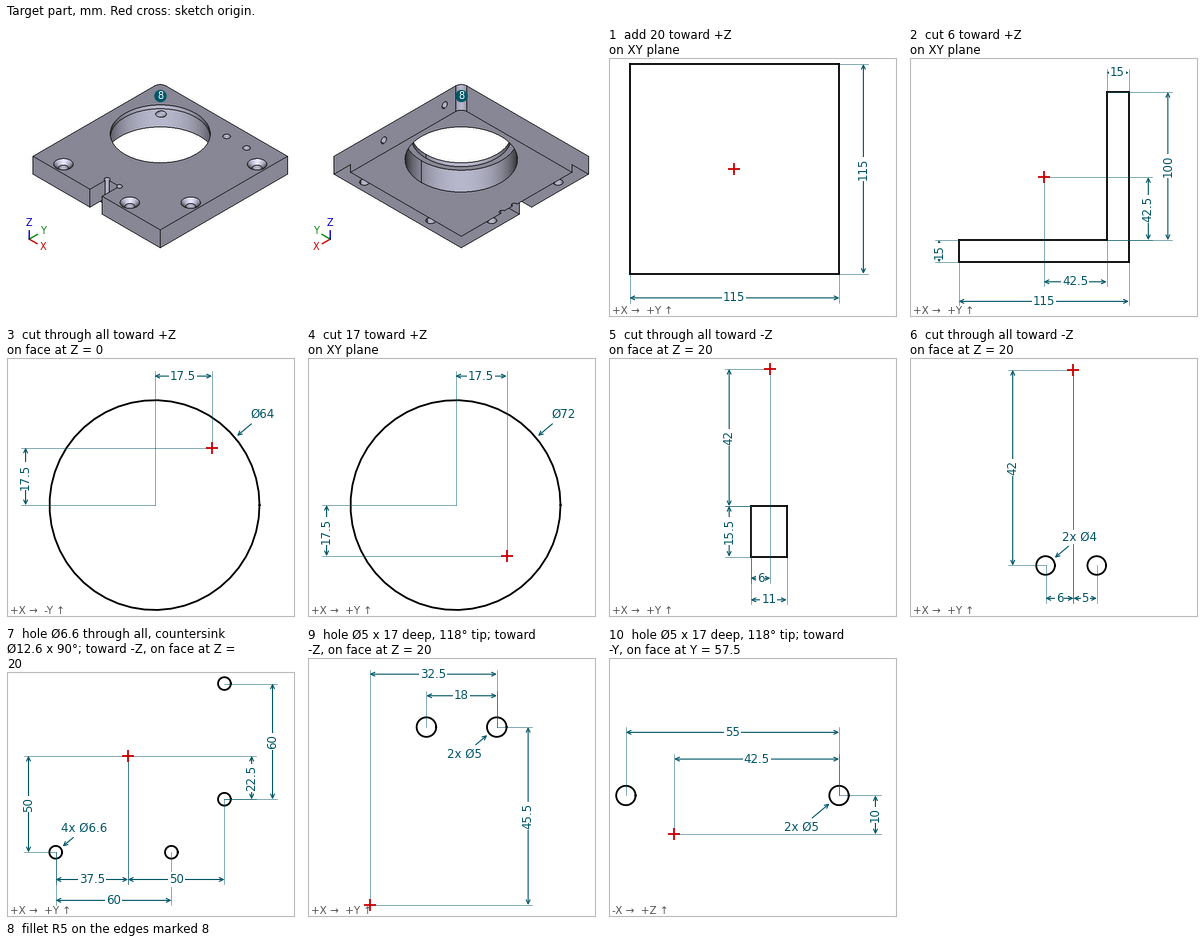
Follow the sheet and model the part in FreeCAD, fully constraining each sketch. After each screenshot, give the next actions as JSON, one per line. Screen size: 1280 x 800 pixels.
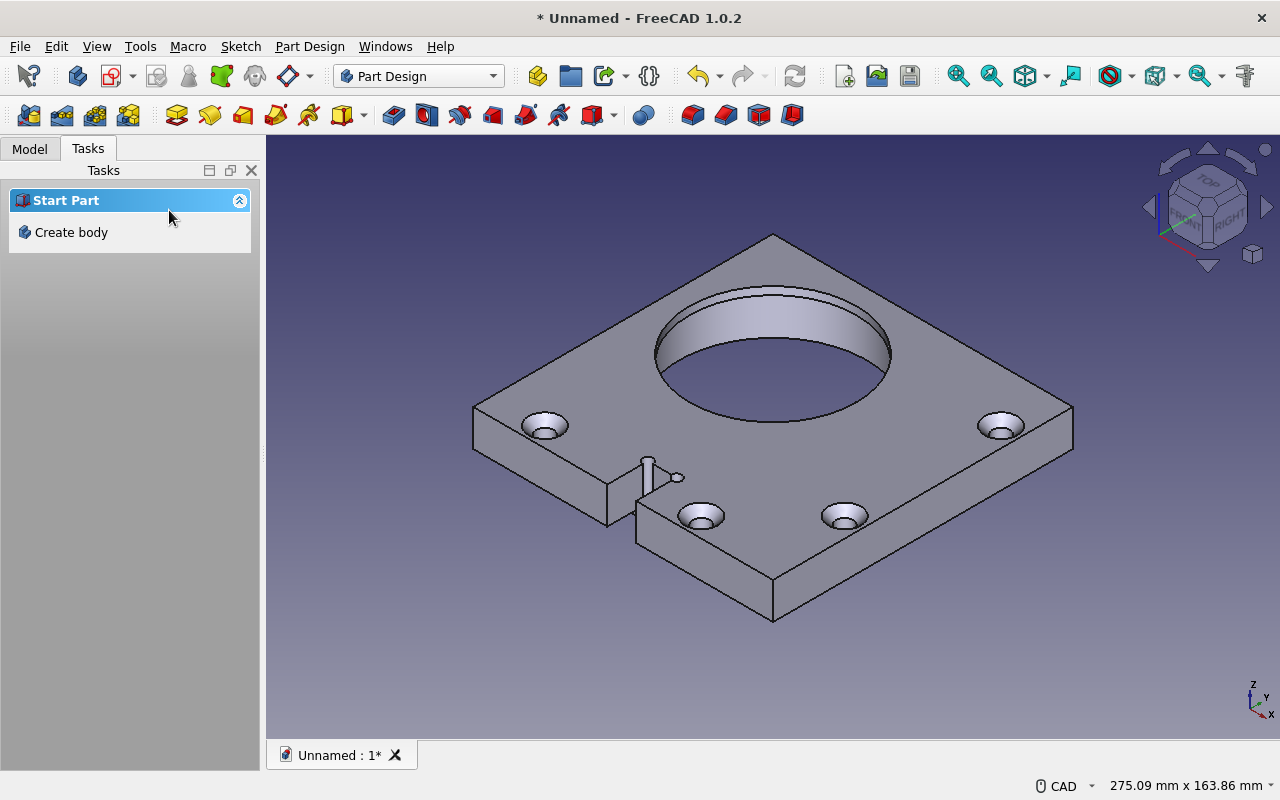
{"action": "key", "text": "2"}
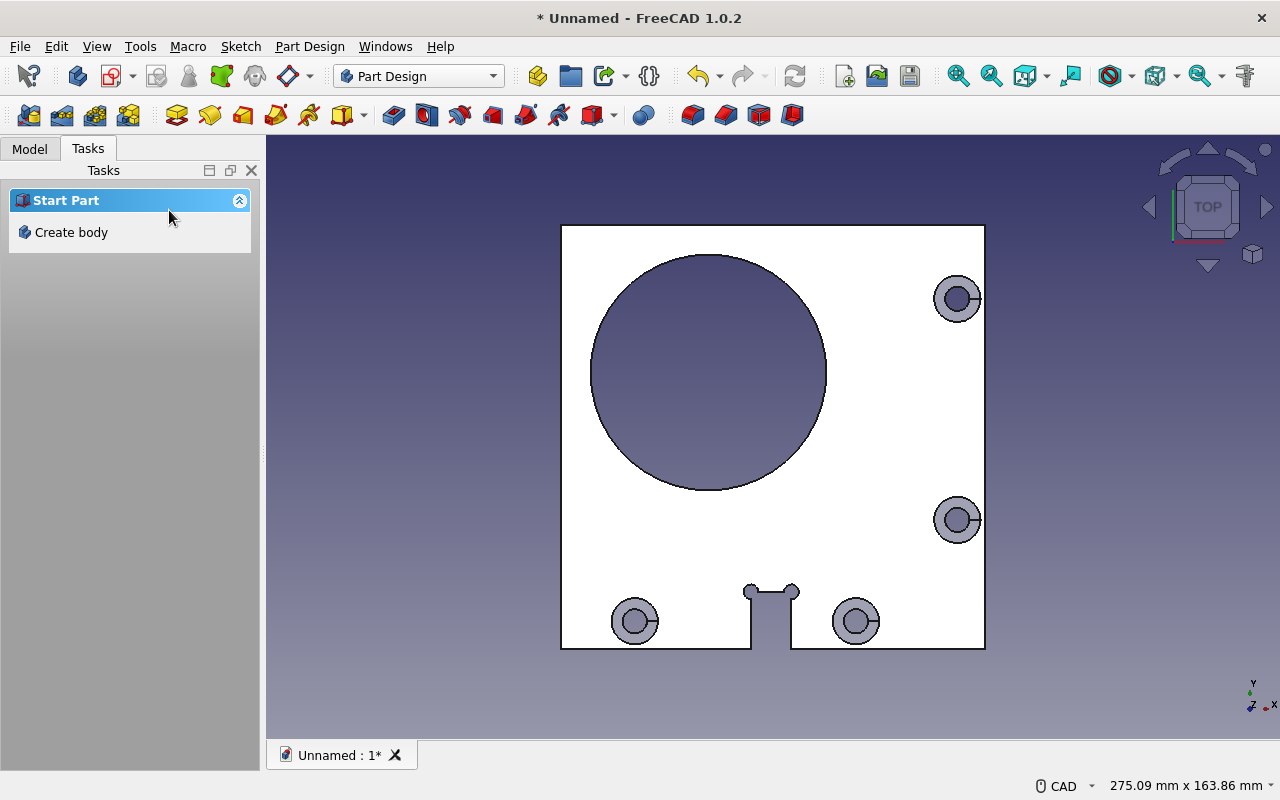
{"action": "key", "text": "0"}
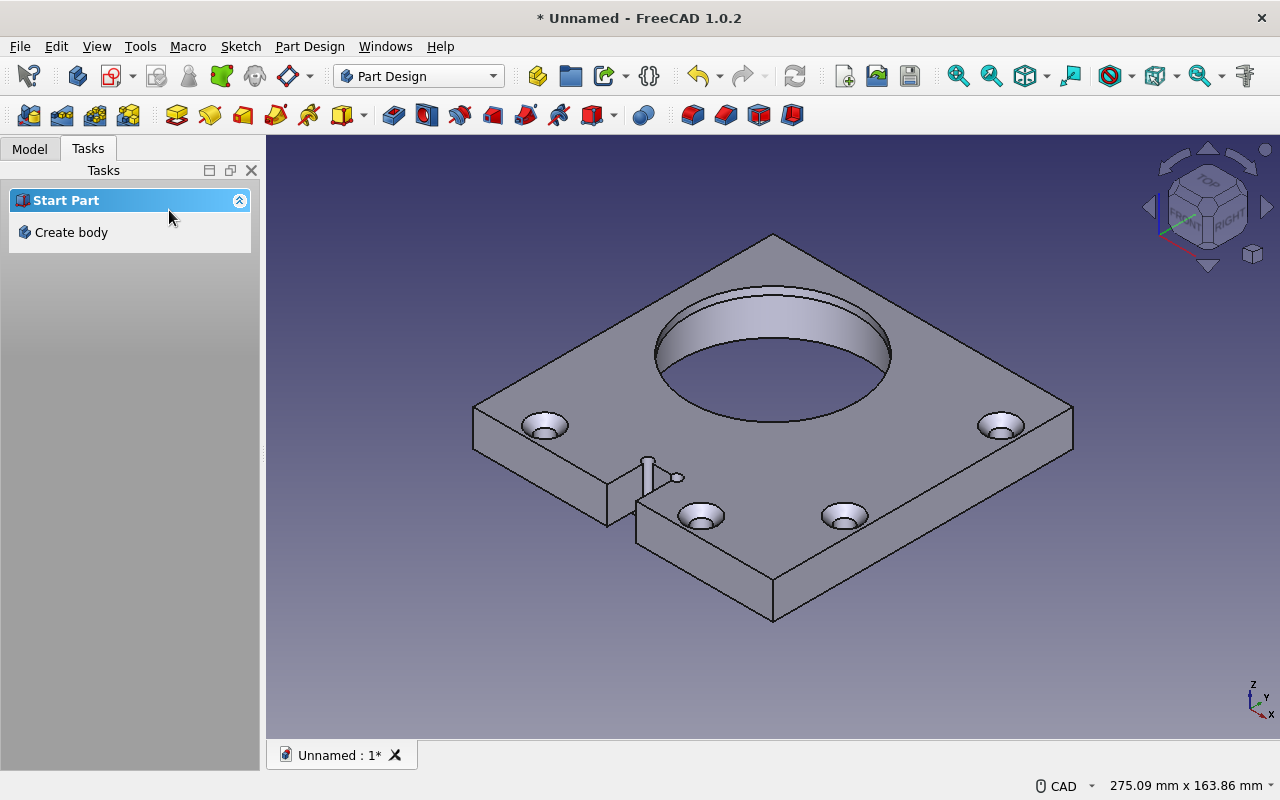
{"action": "key", "text": "1"}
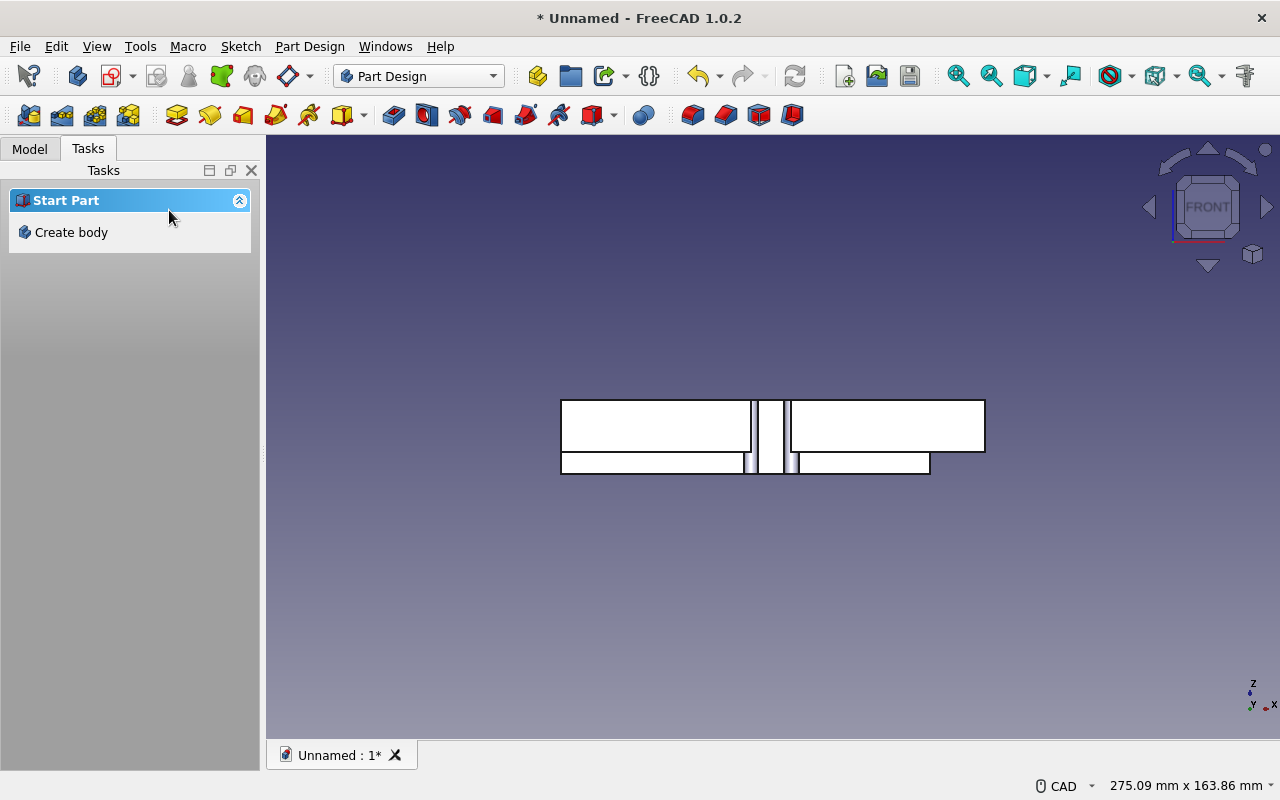
{"action": "key", "text": "v f"}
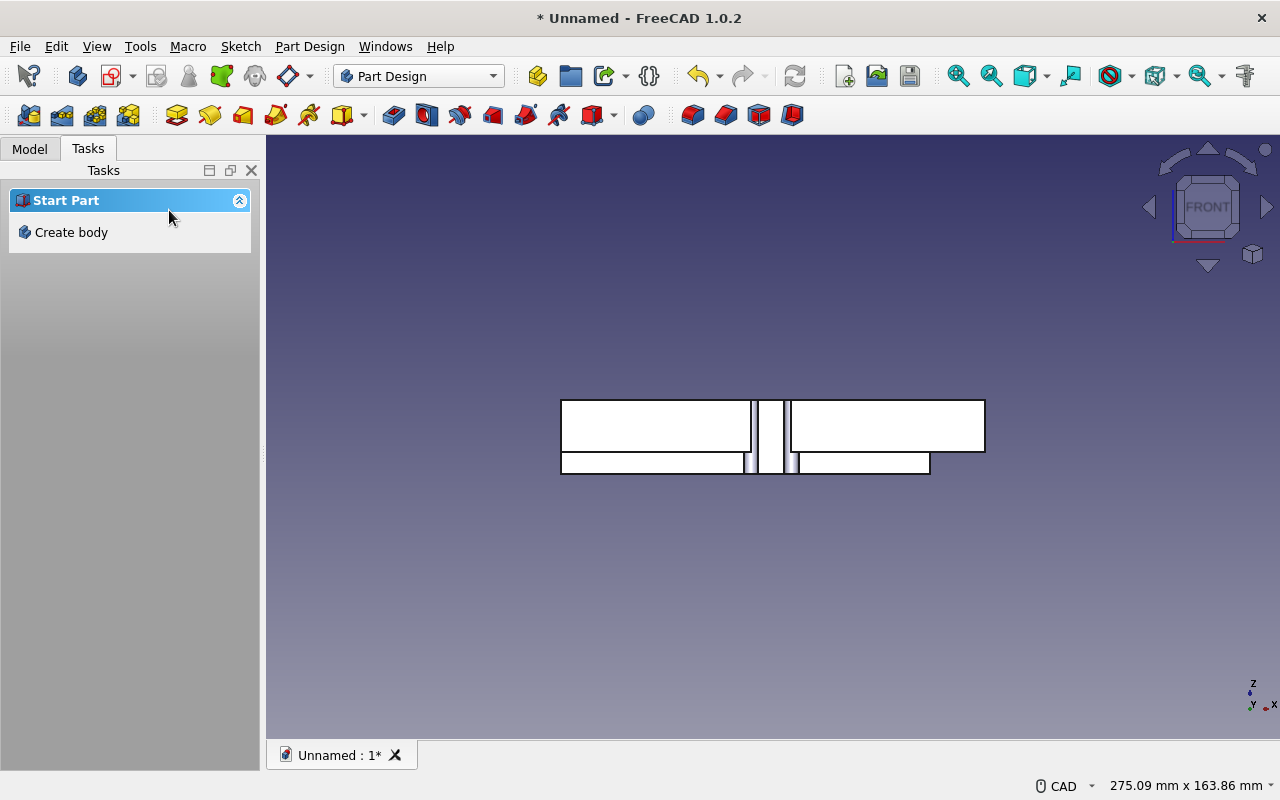
{"action": "key", "text": "3"}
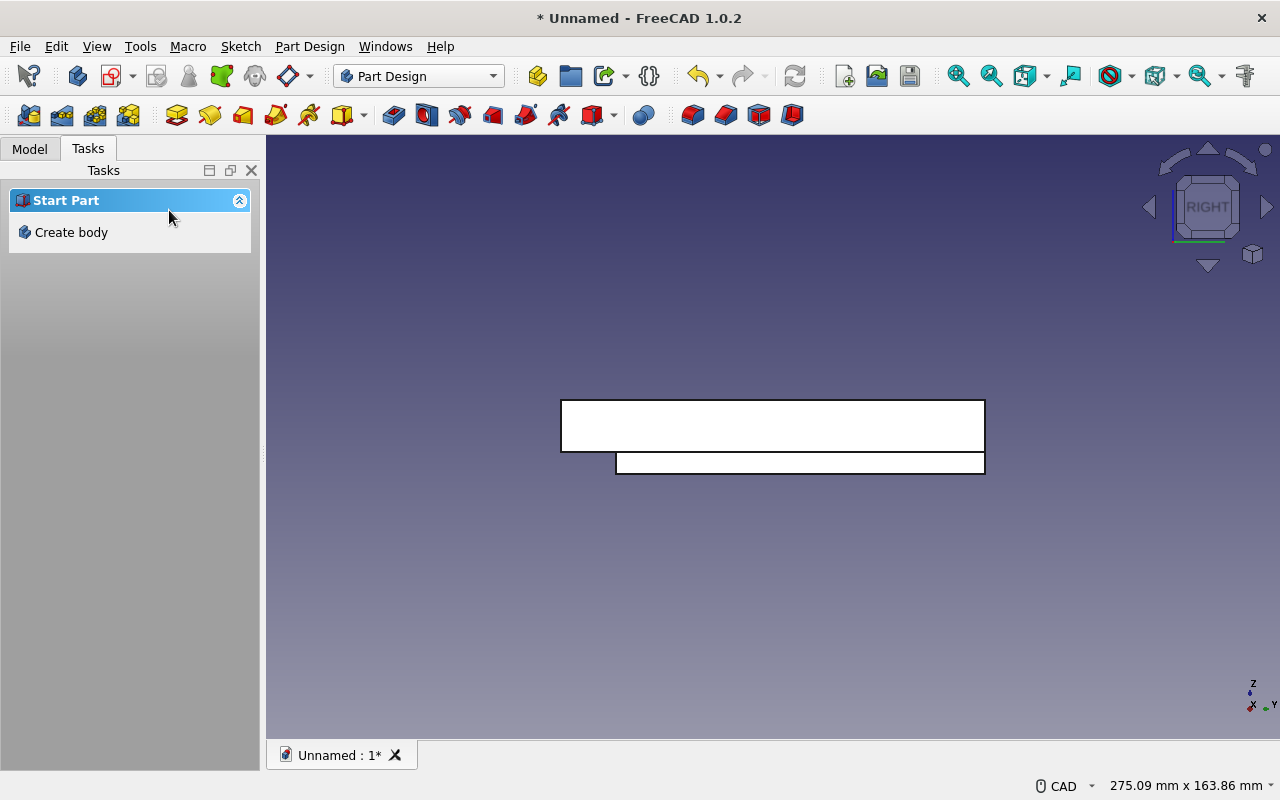
{"action": "key", "text": "v f"}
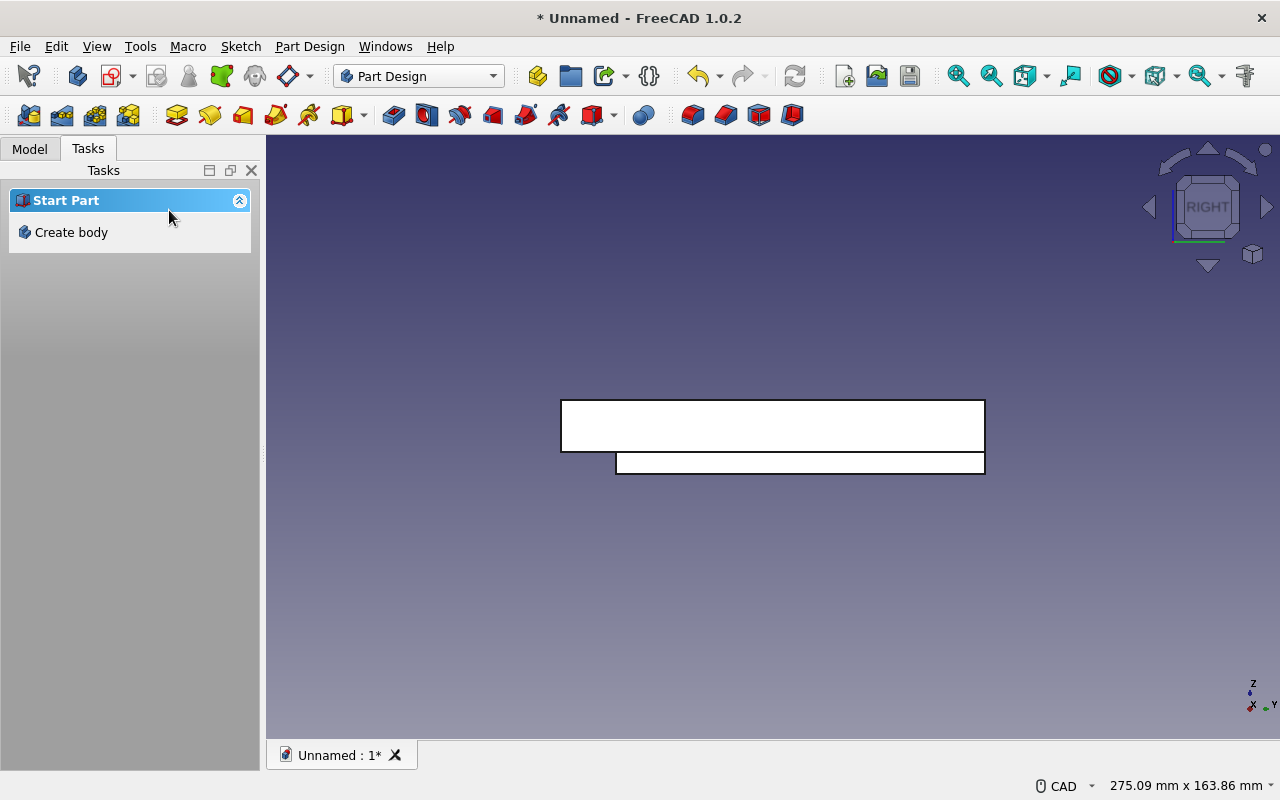
{"action": "key", "text": "5"}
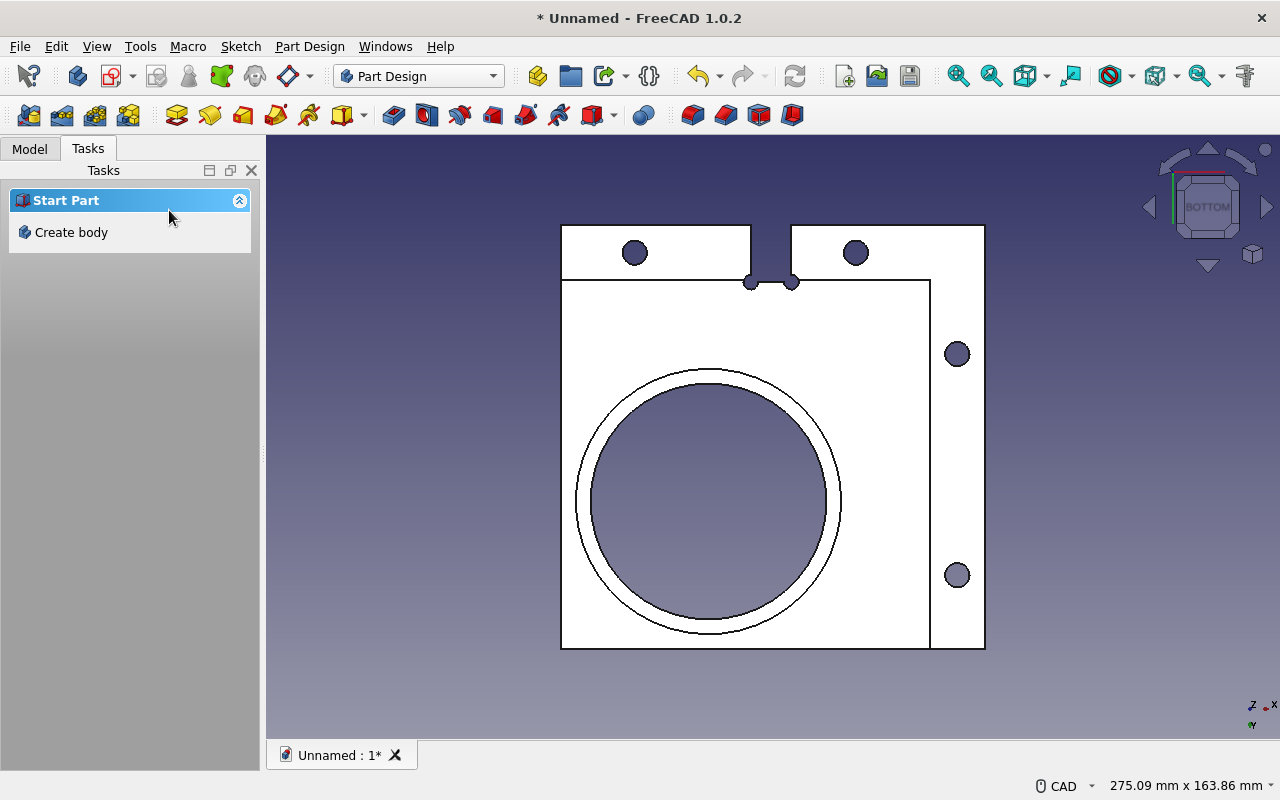
{"action": "key", "text": "4"}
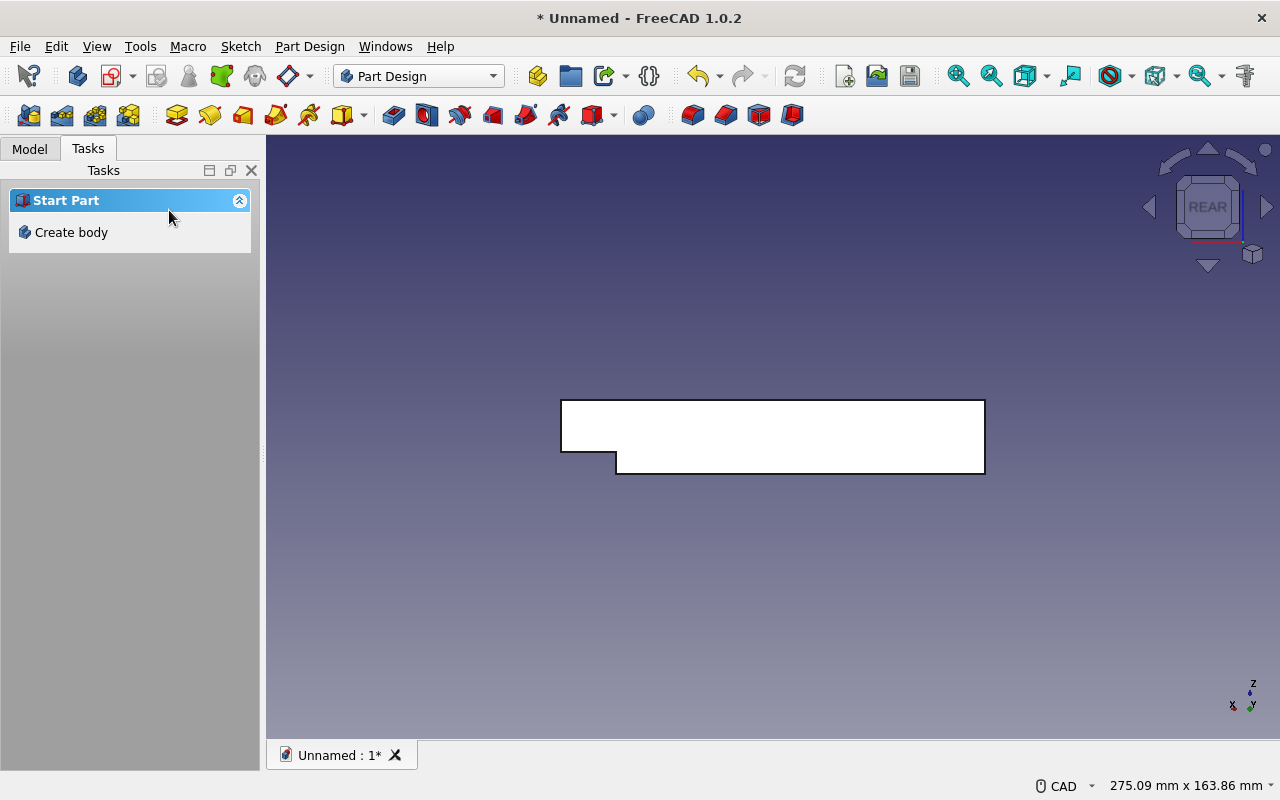
{"action": "key", "text": "v f"}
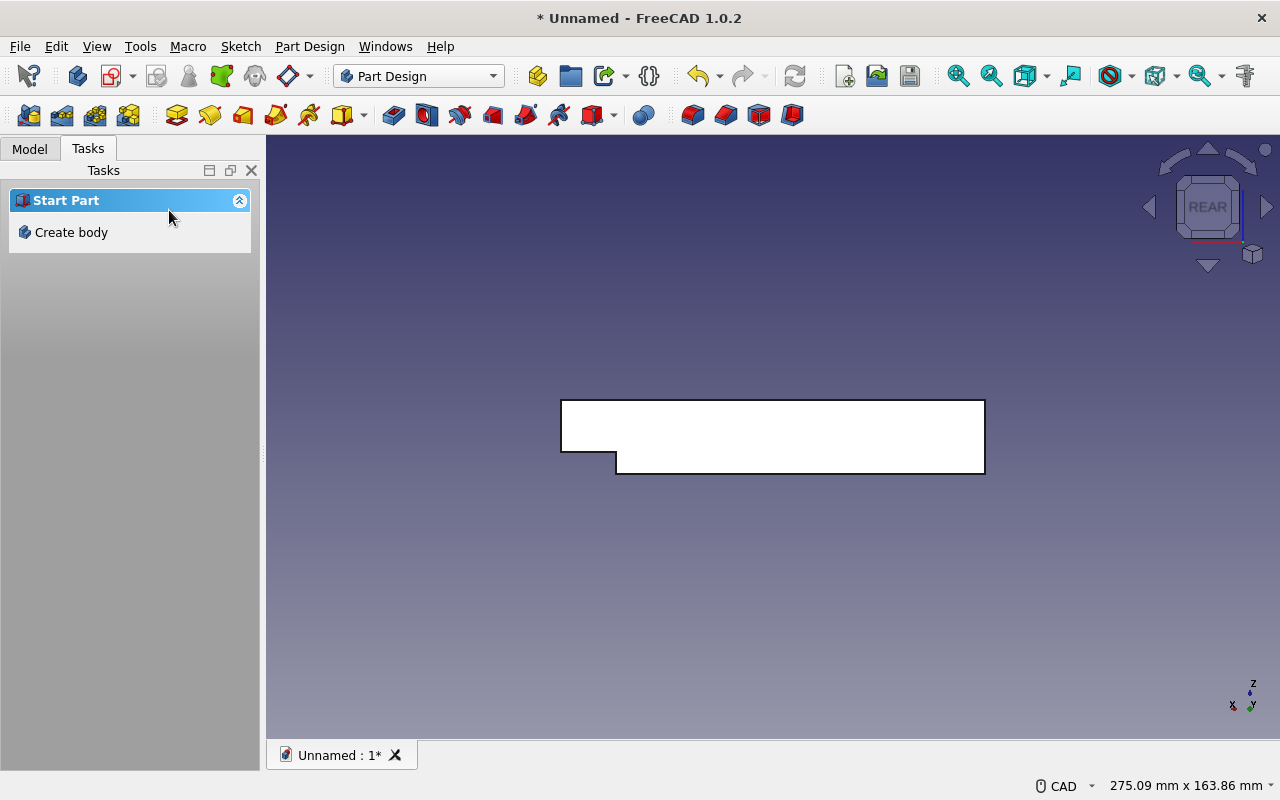
{"action": "left_click", "coordinate": [985, 436]}